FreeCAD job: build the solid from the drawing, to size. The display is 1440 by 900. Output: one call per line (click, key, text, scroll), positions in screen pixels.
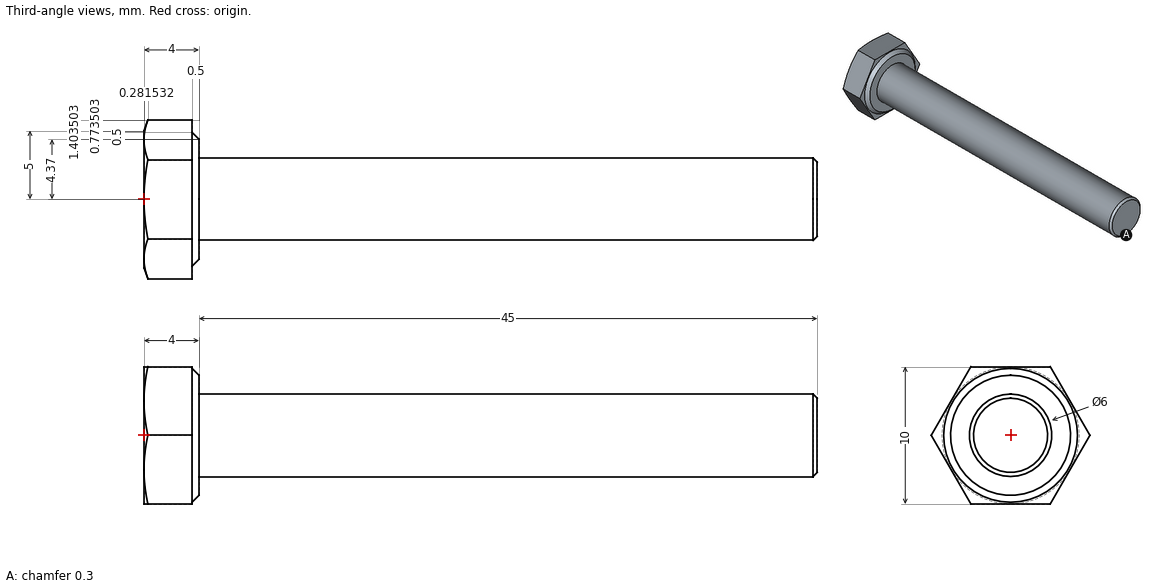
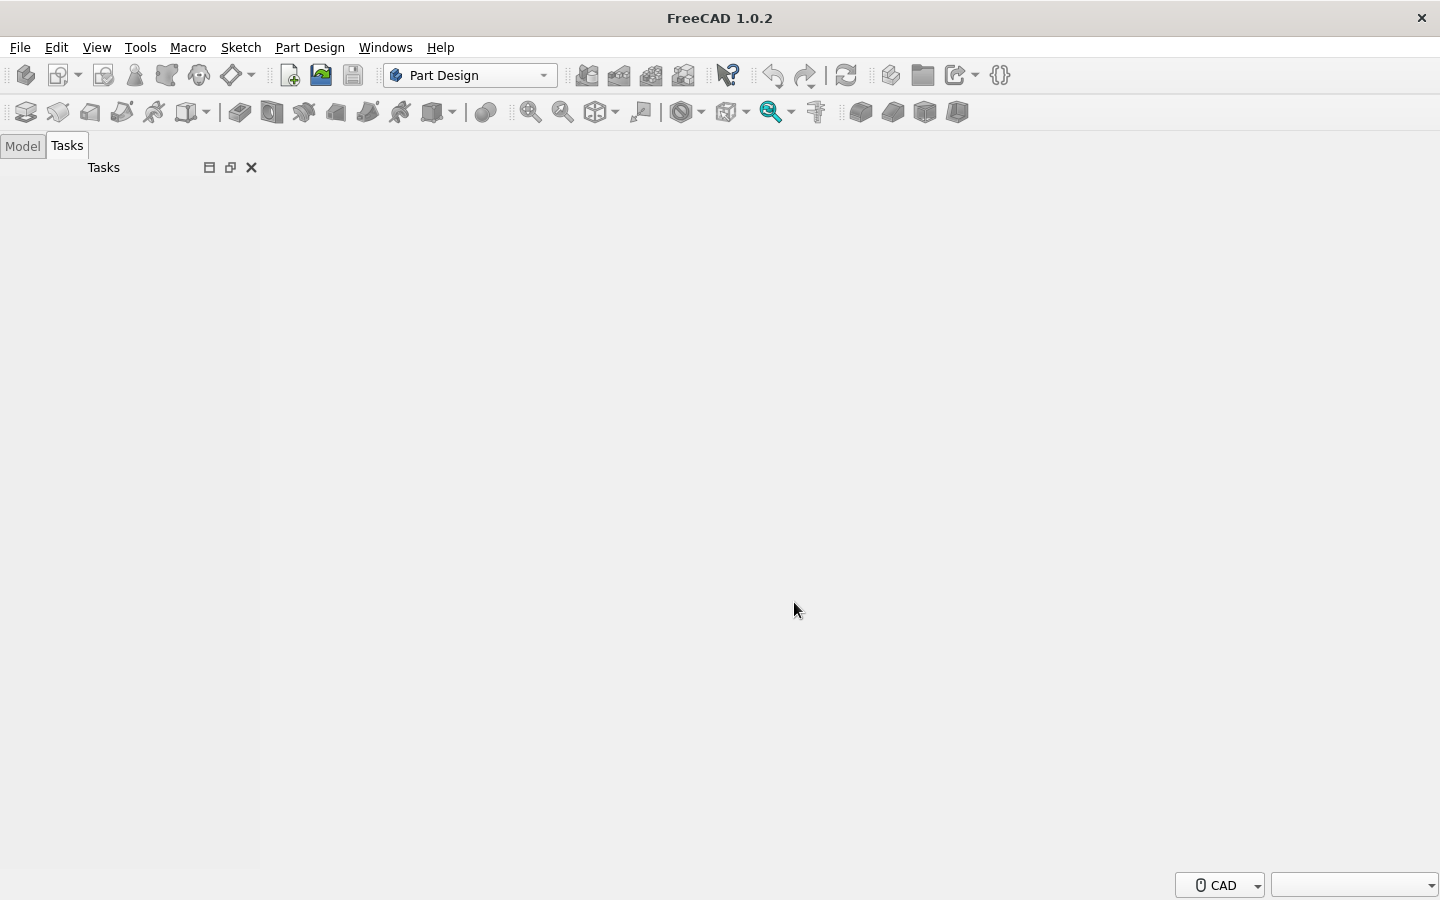
click(290, 76)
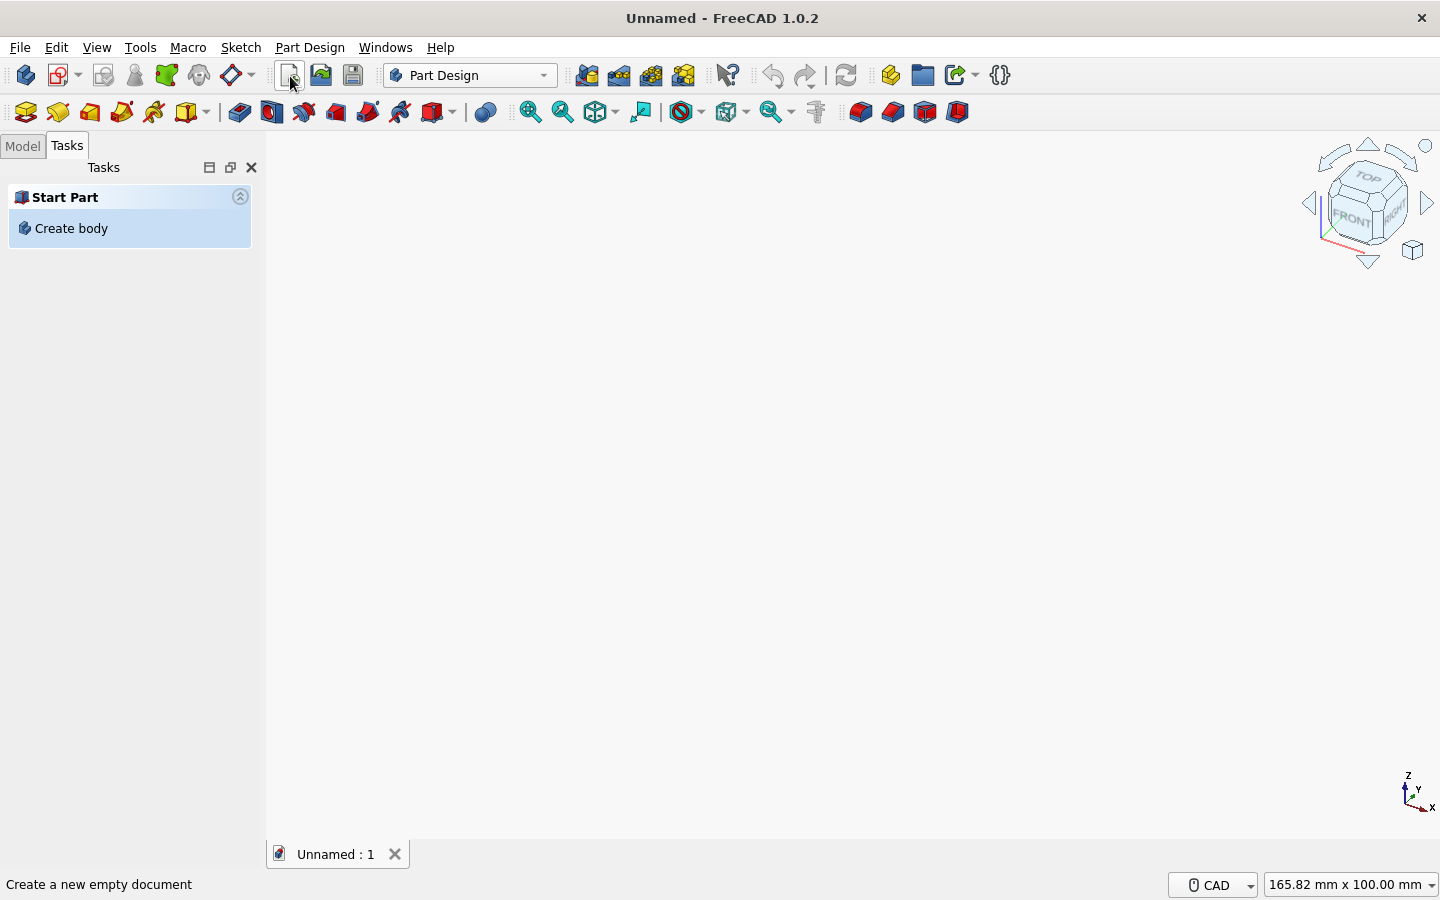
click(58, 76)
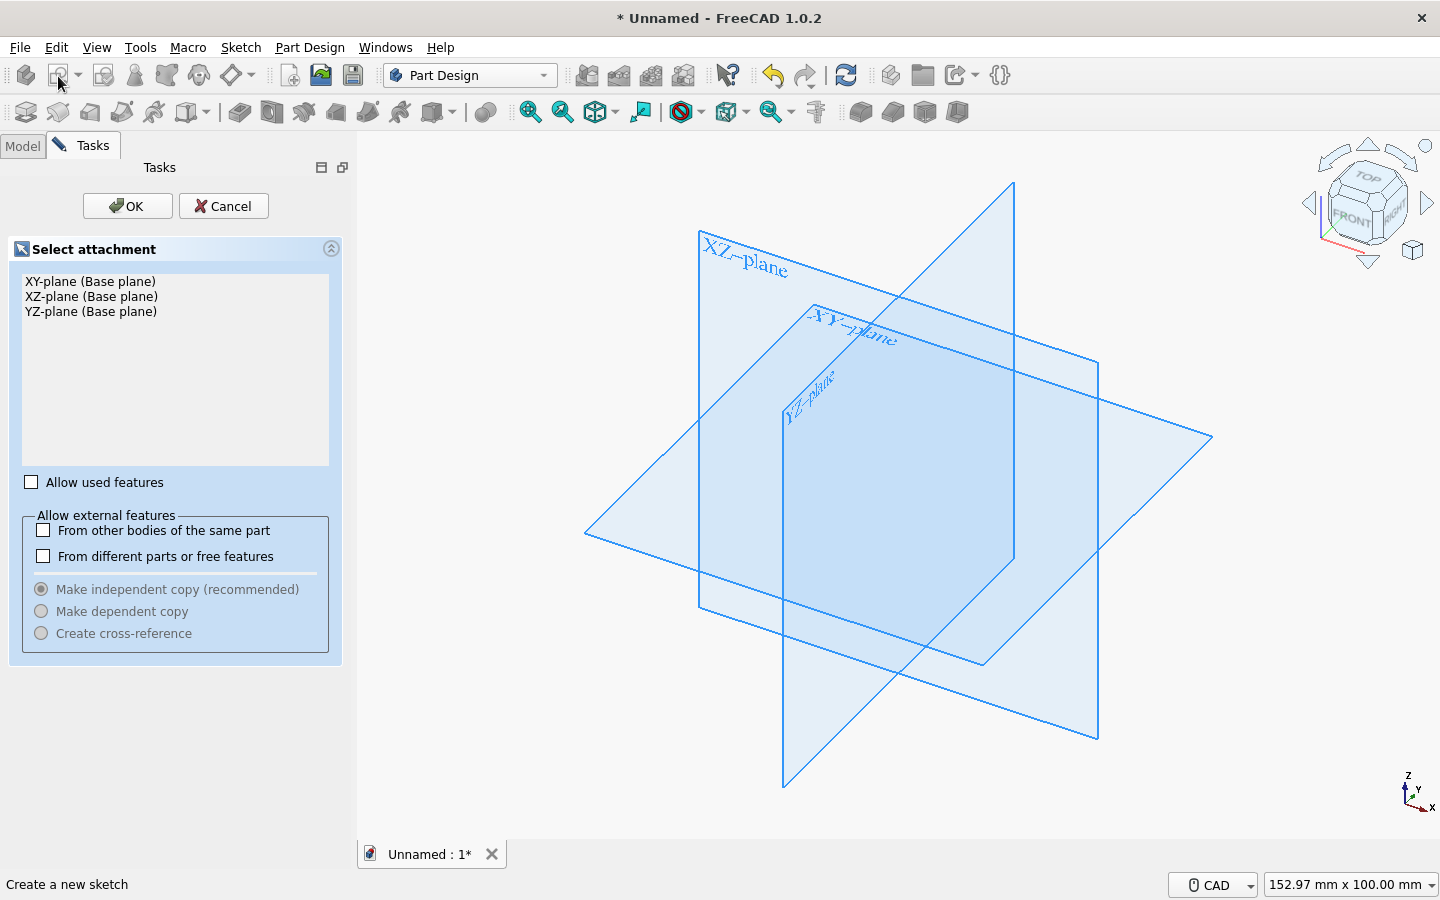
click(82, 312)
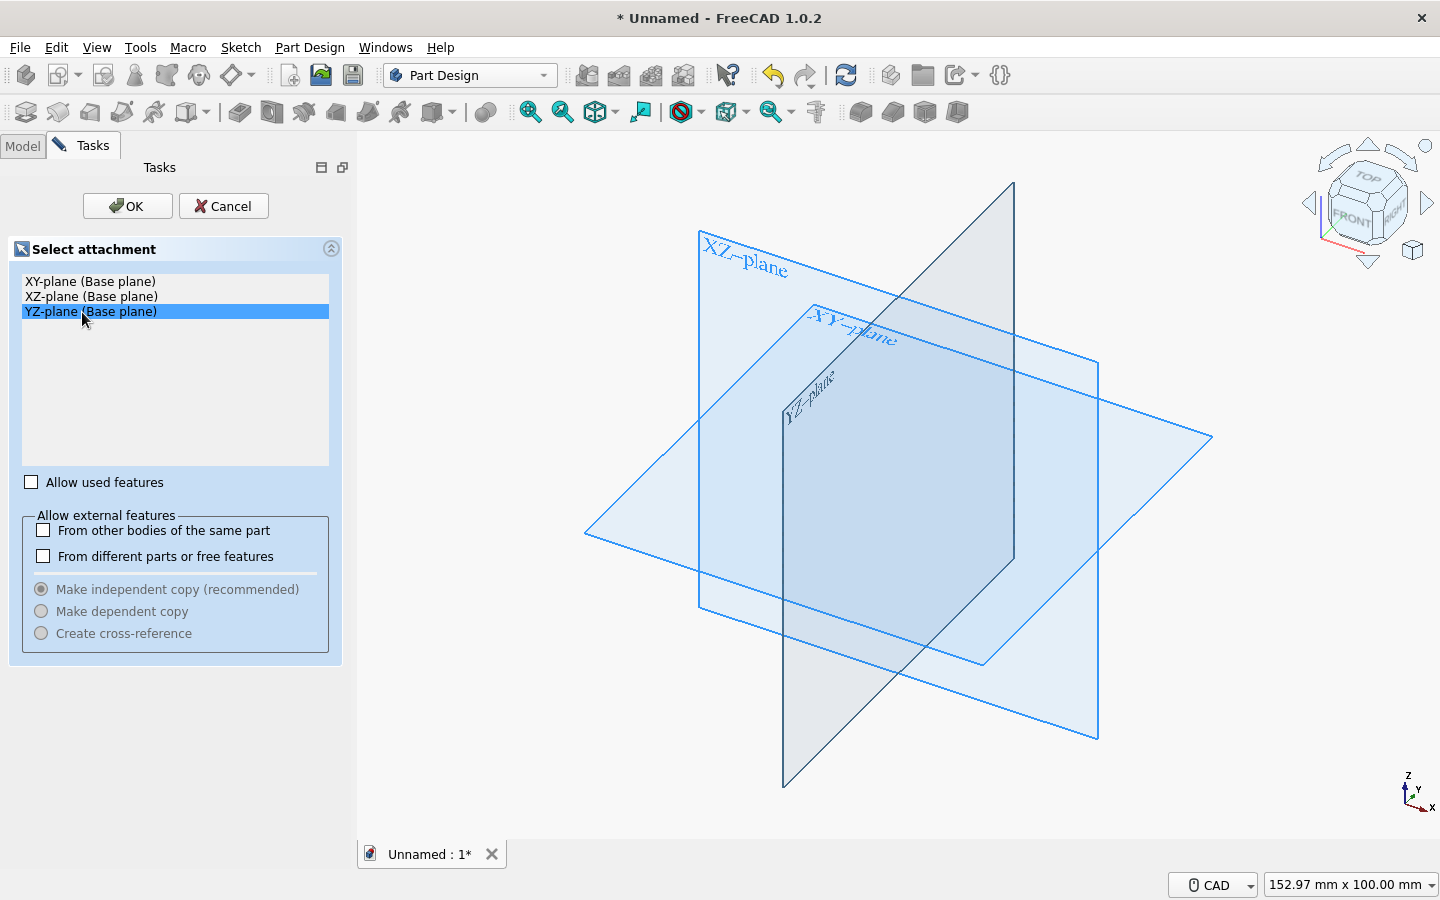
click(128, 206)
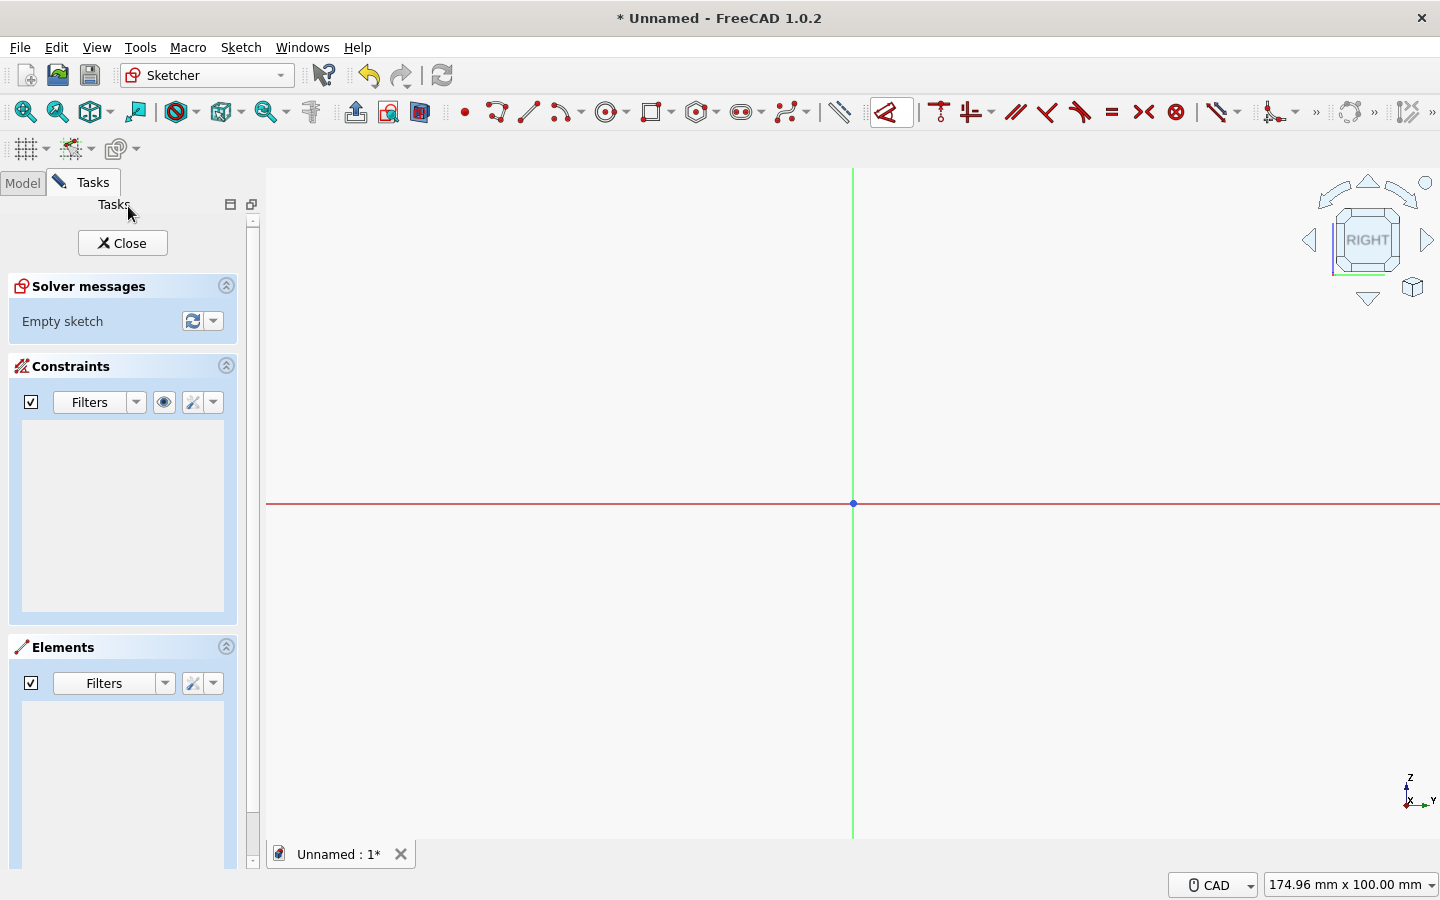
scroll(867, 504, up, 9)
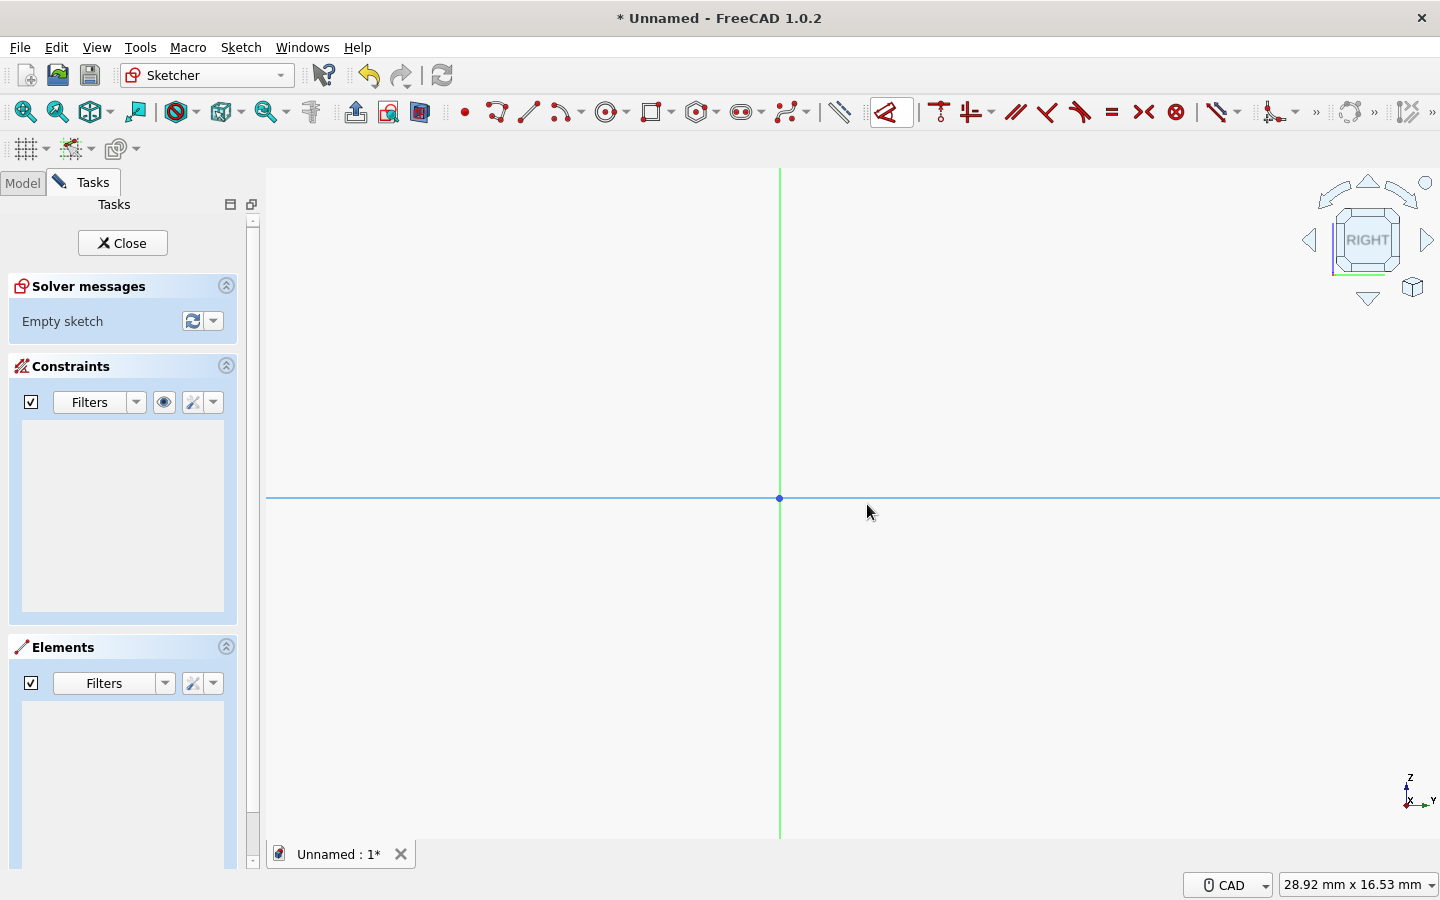
click(696, 112)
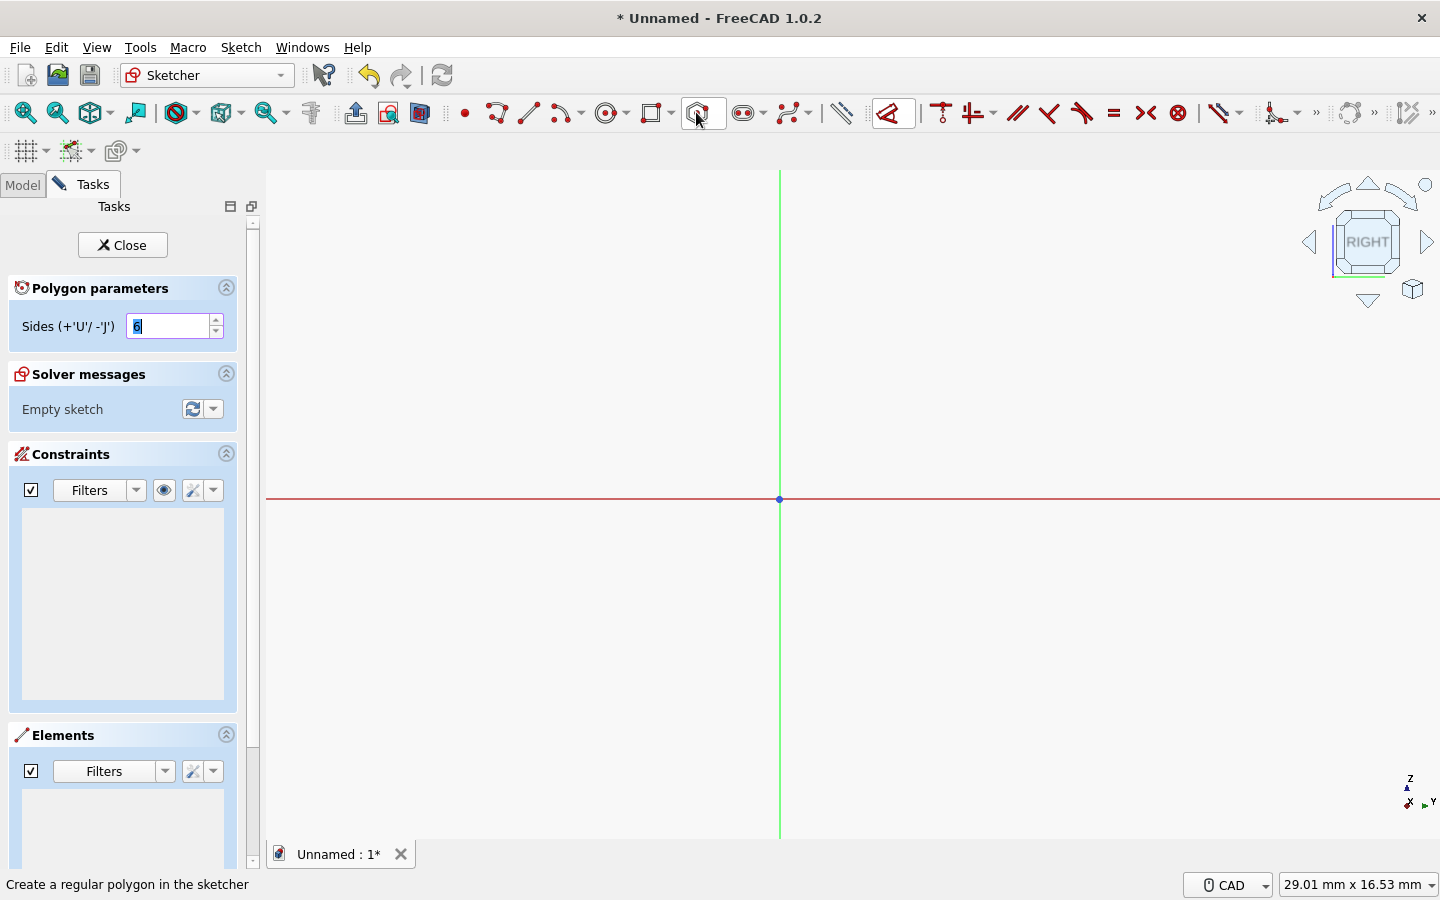
click(780, 499)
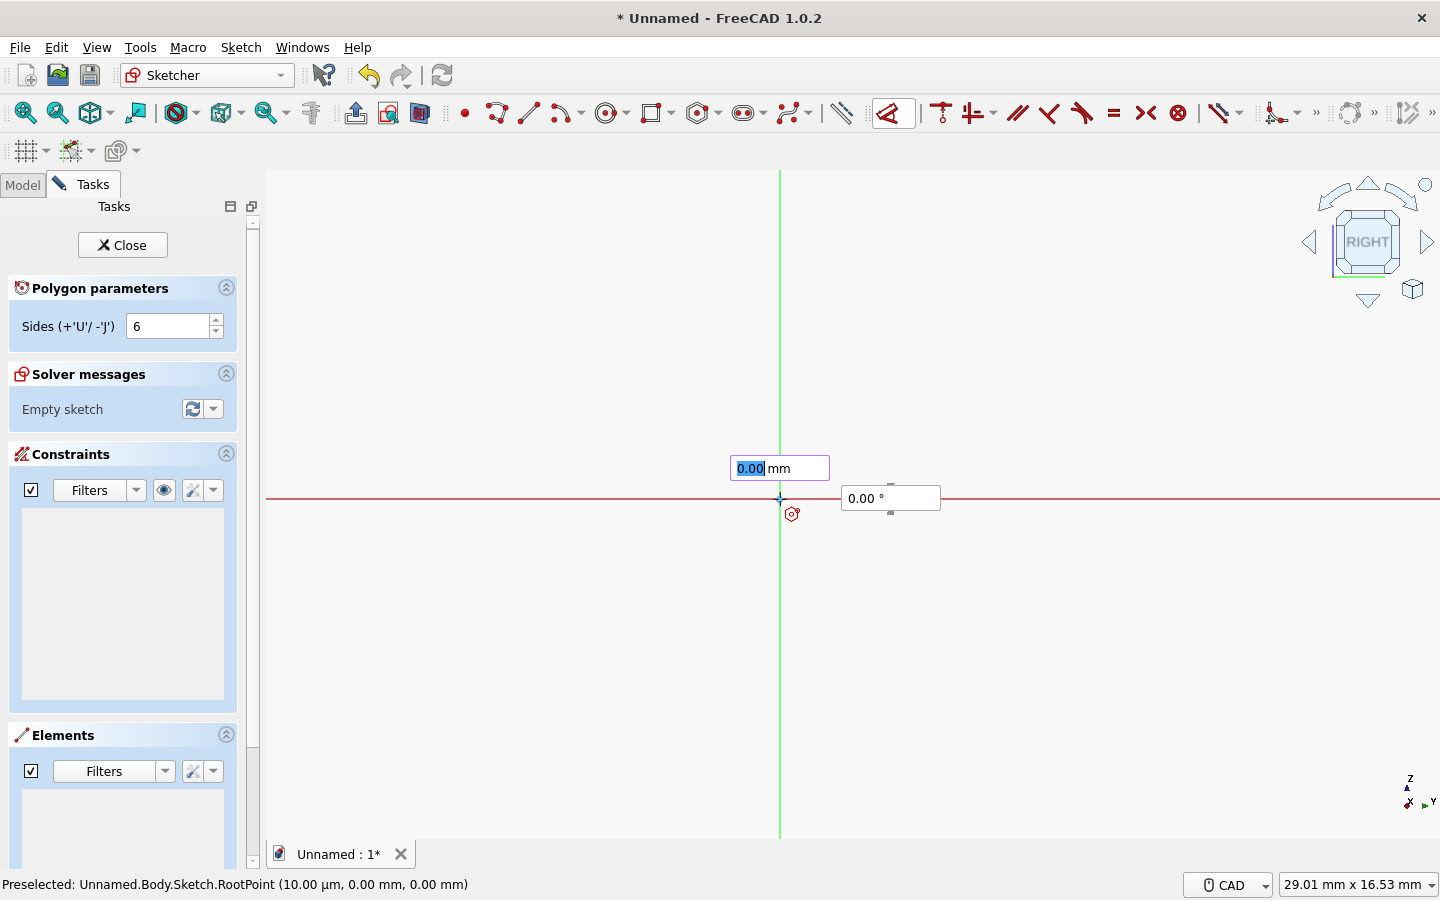
click(546, 499)
right_click(546, 499)